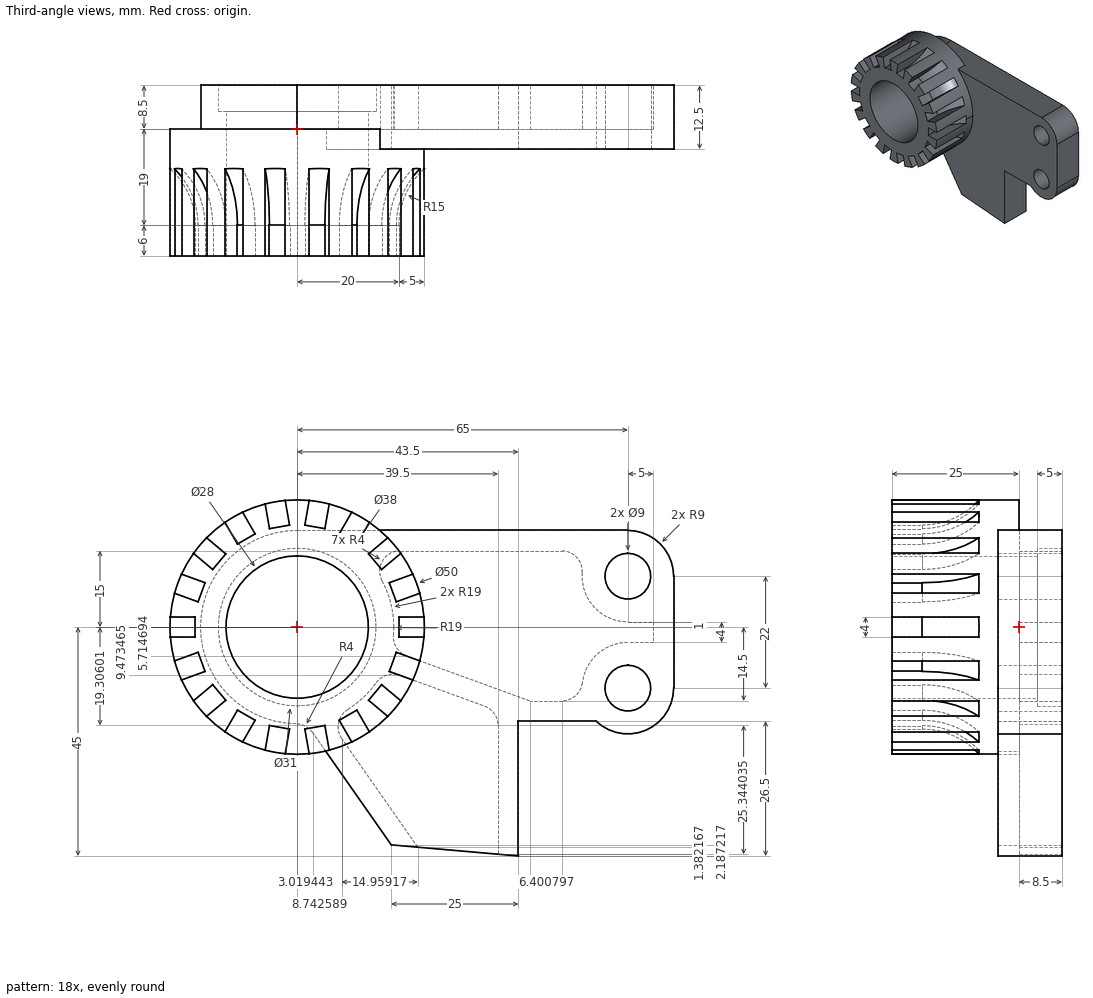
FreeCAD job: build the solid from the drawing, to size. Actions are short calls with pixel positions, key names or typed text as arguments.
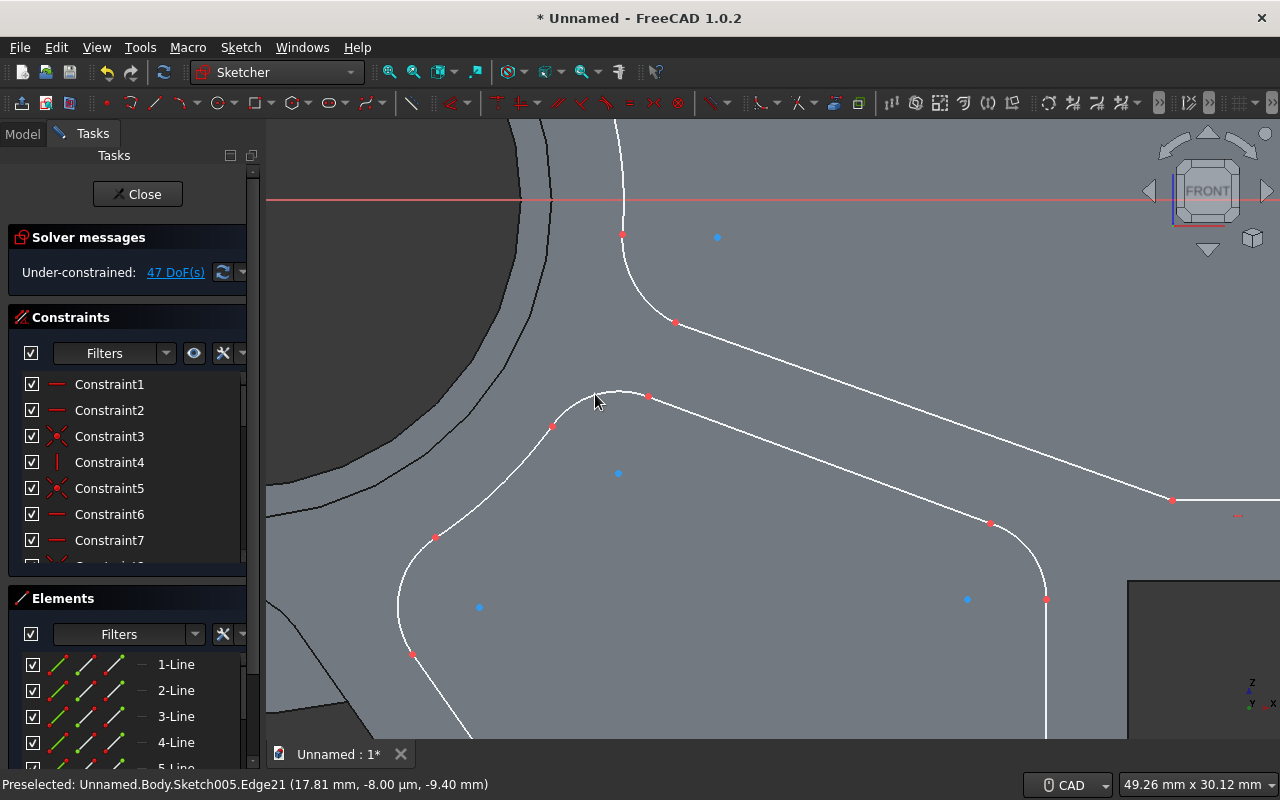
scroll(597, 396, down, 6)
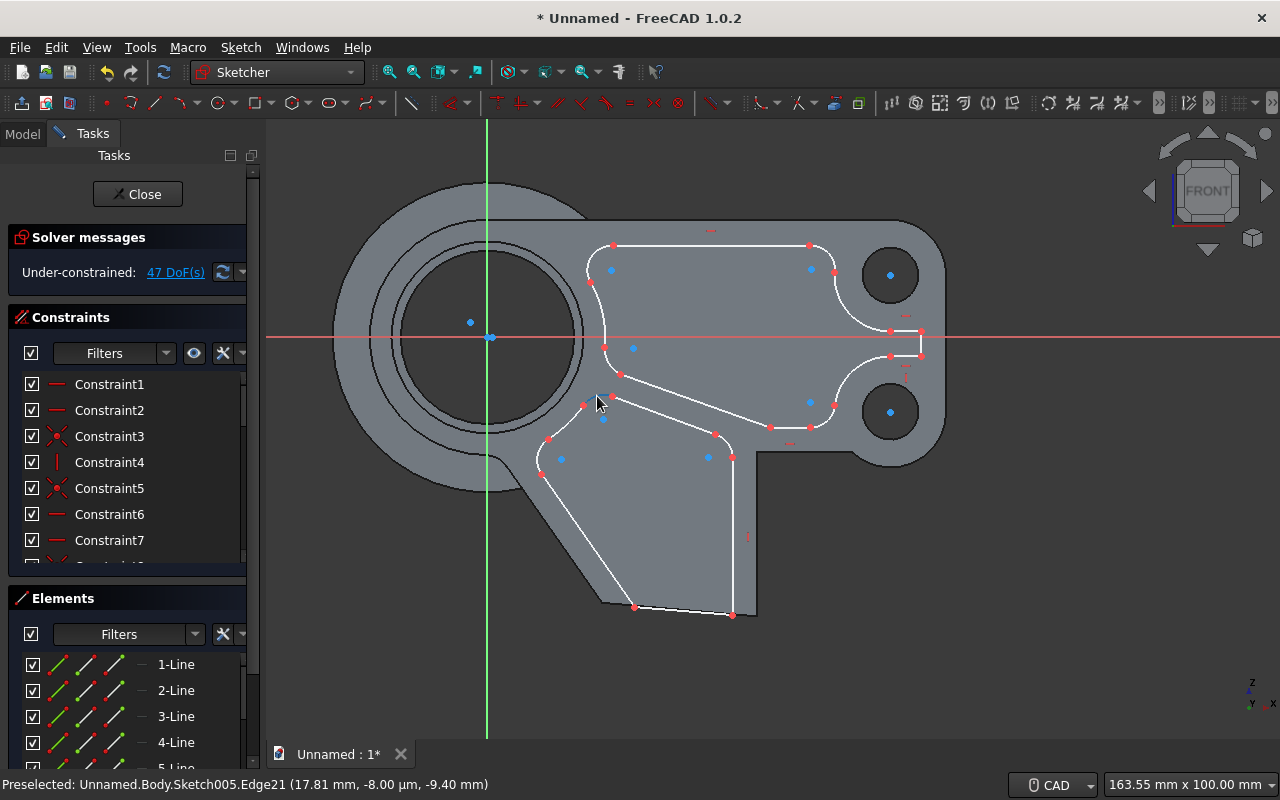
click(672, 246)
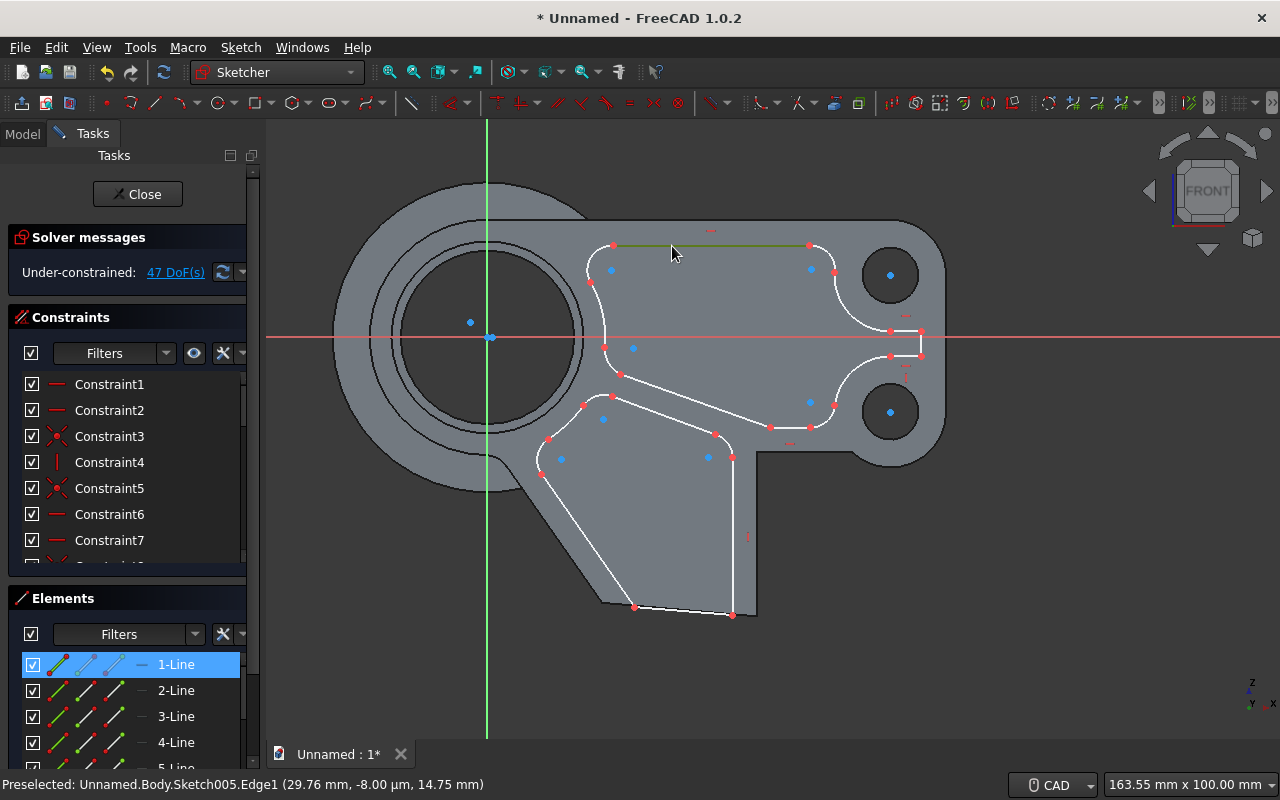
click(833, 260)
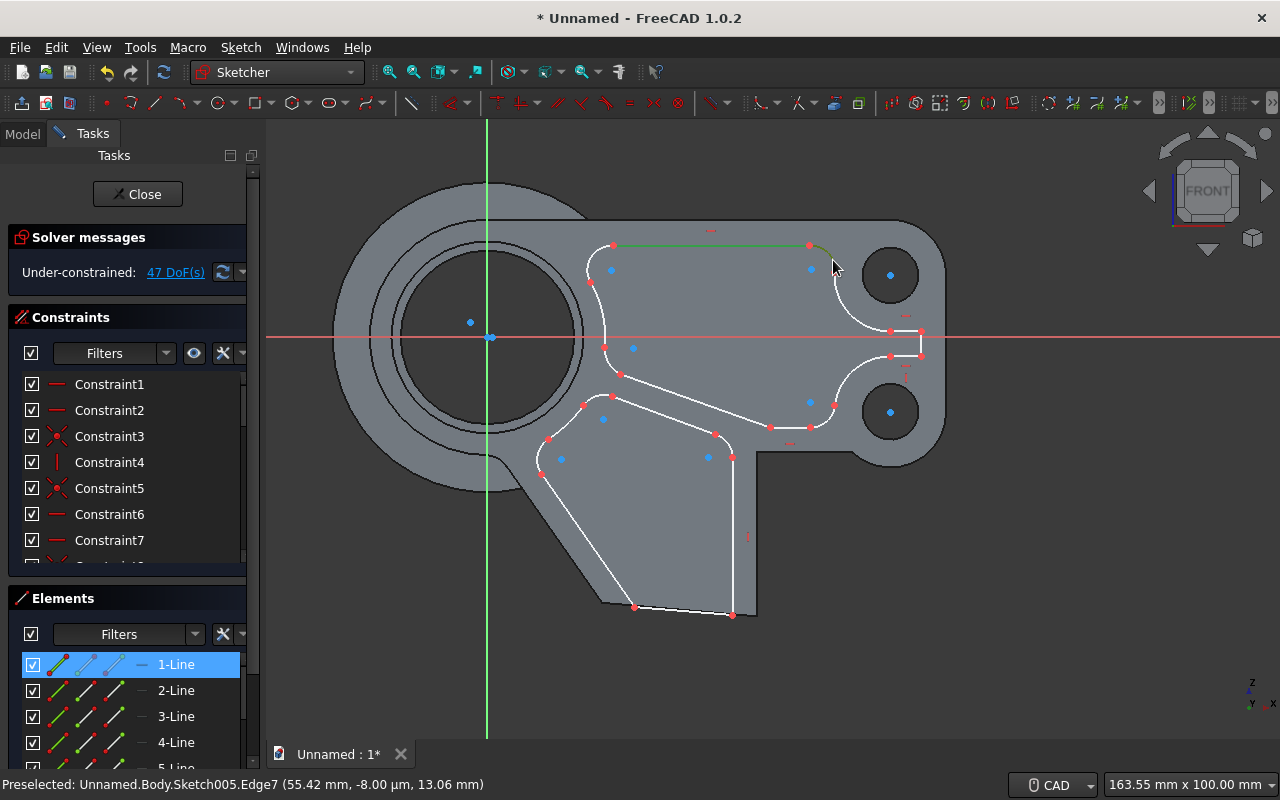
click(606, 104)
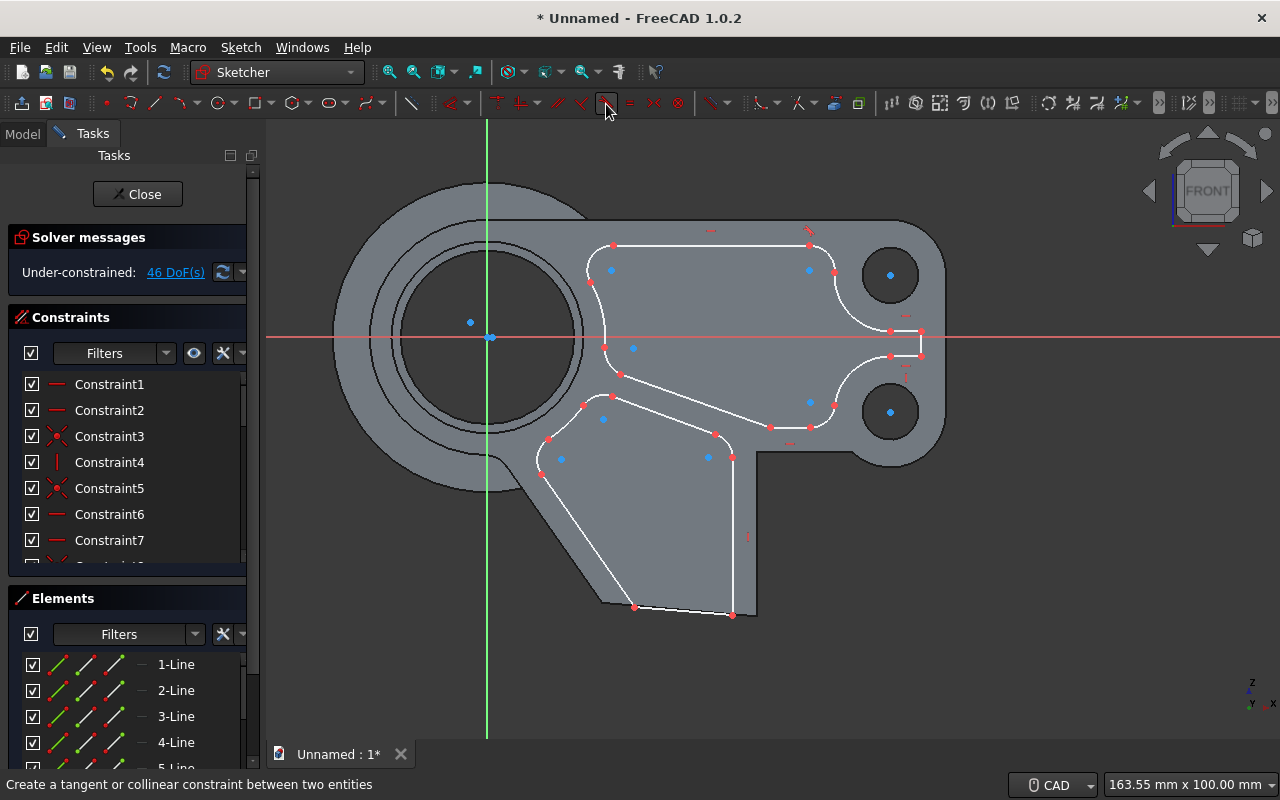
click(672, 246)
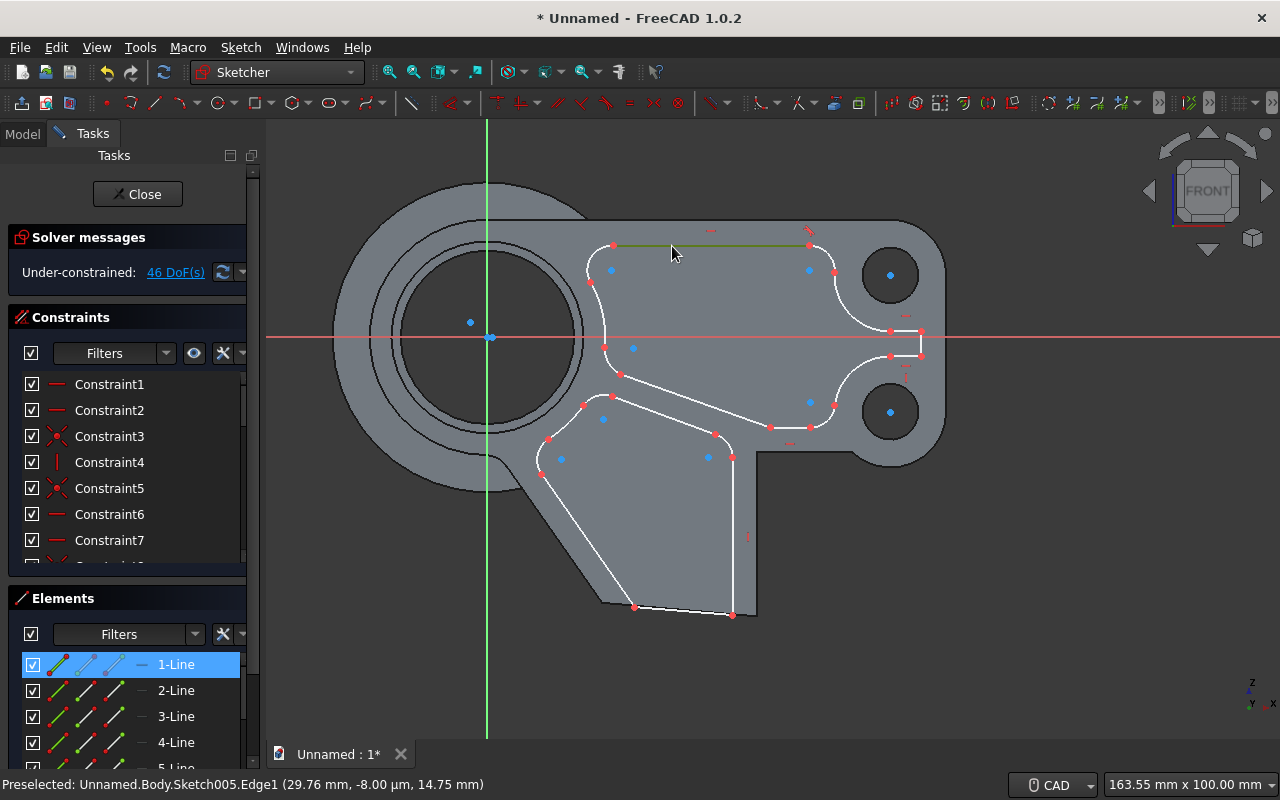
click(598, 250)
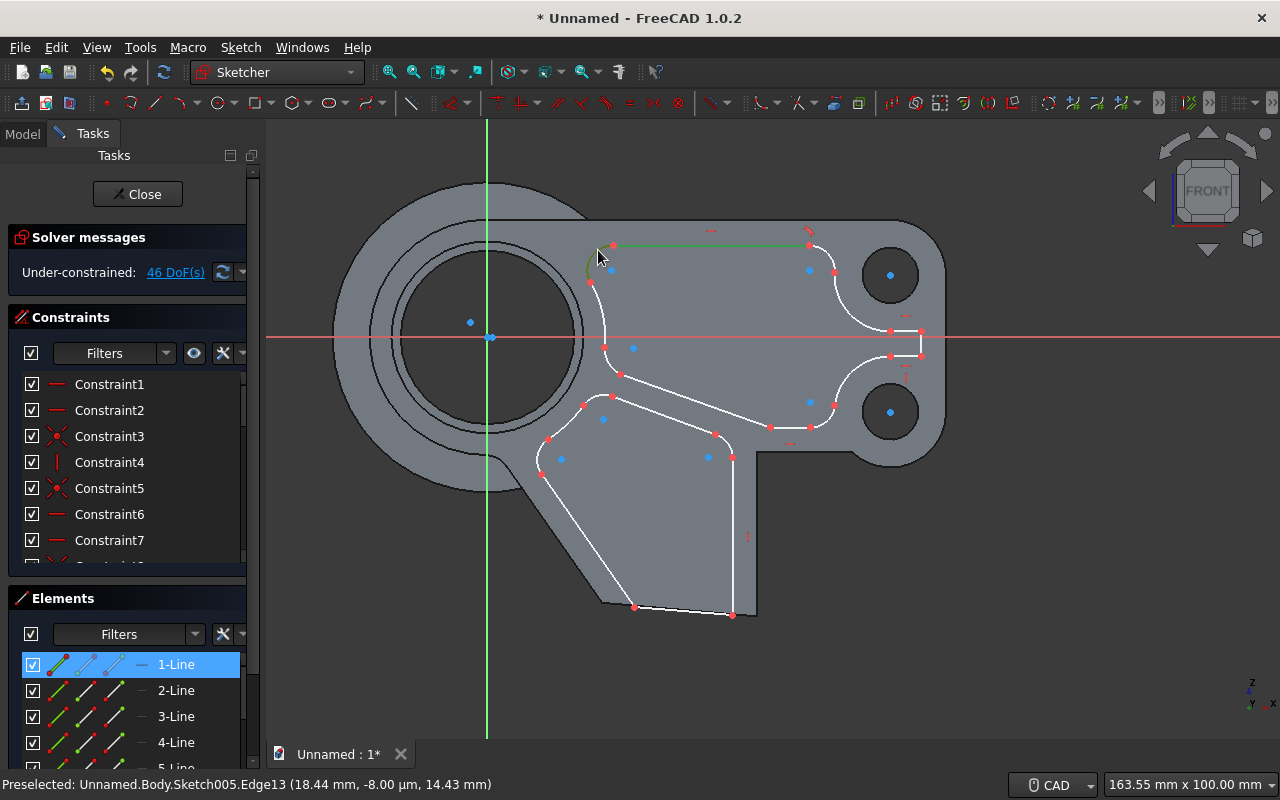
click(606, 104)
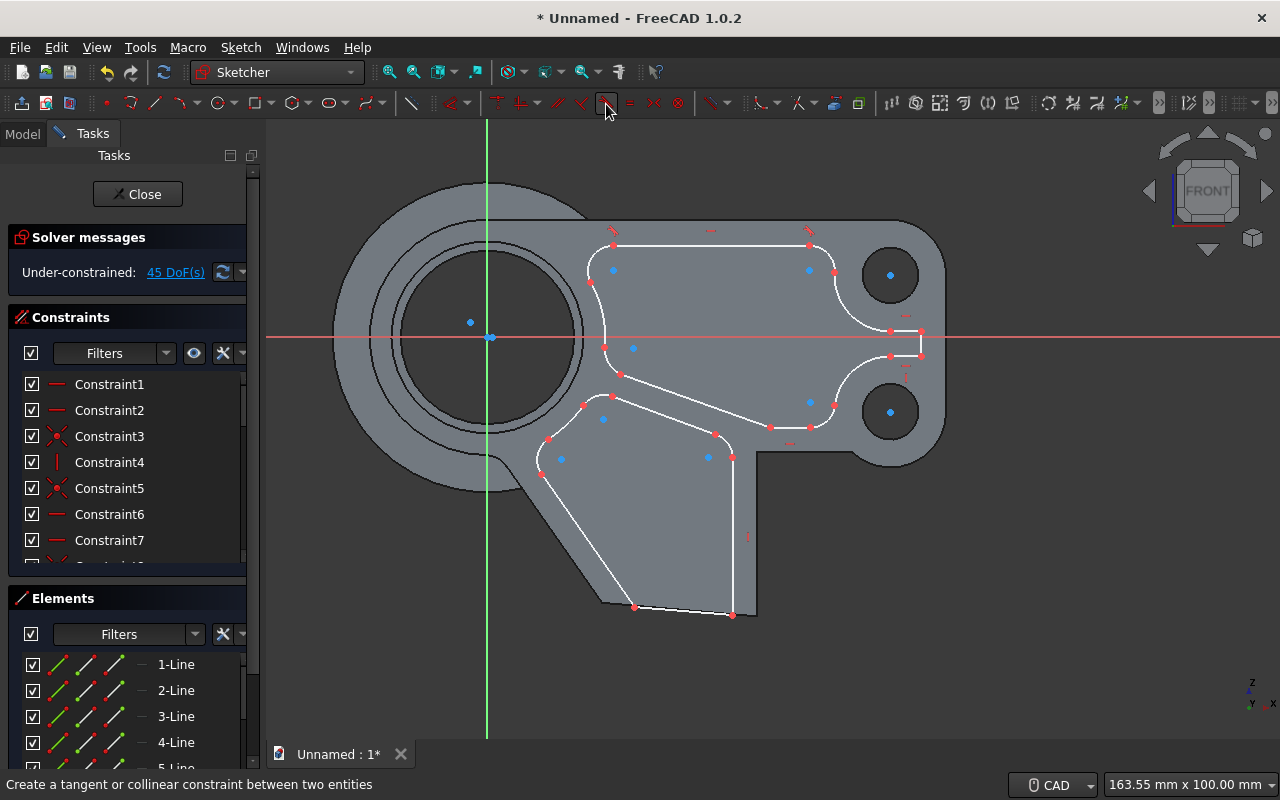
scroll(900, 331, up, 5)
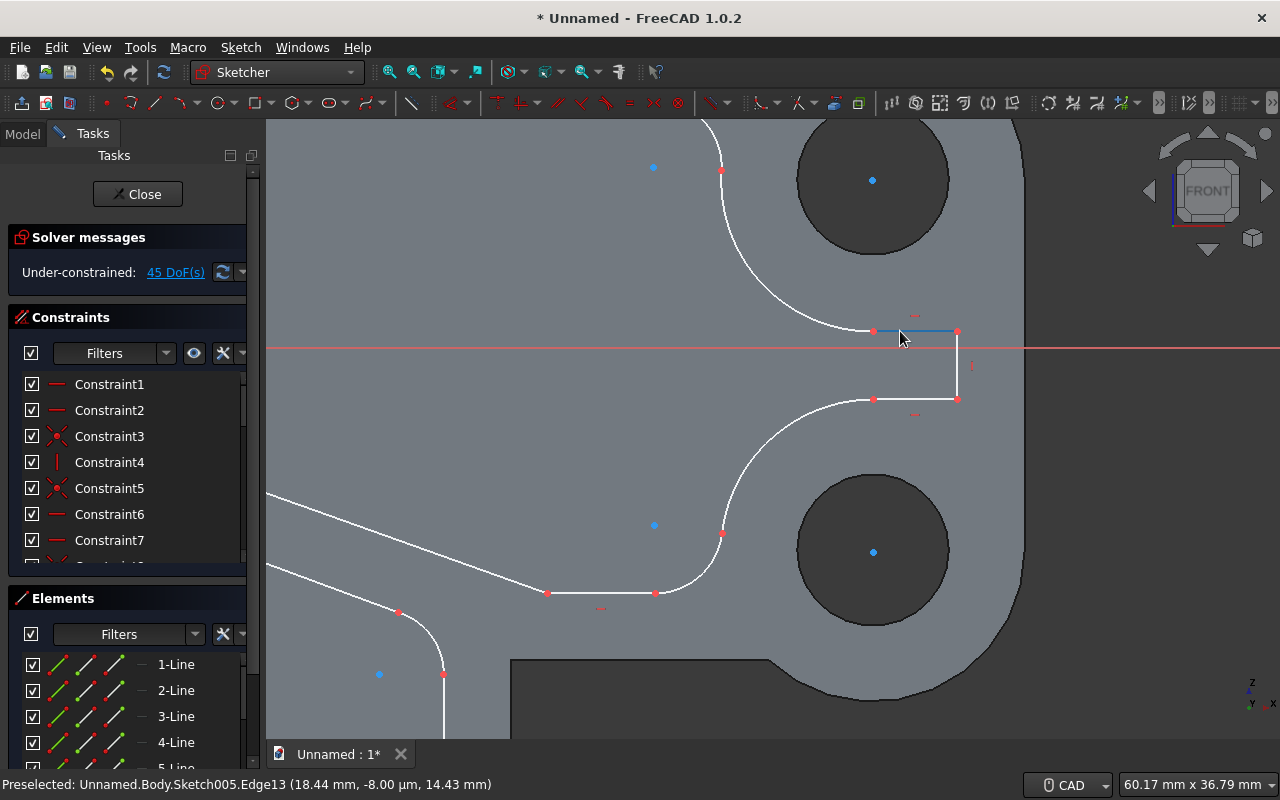
click(899, 331)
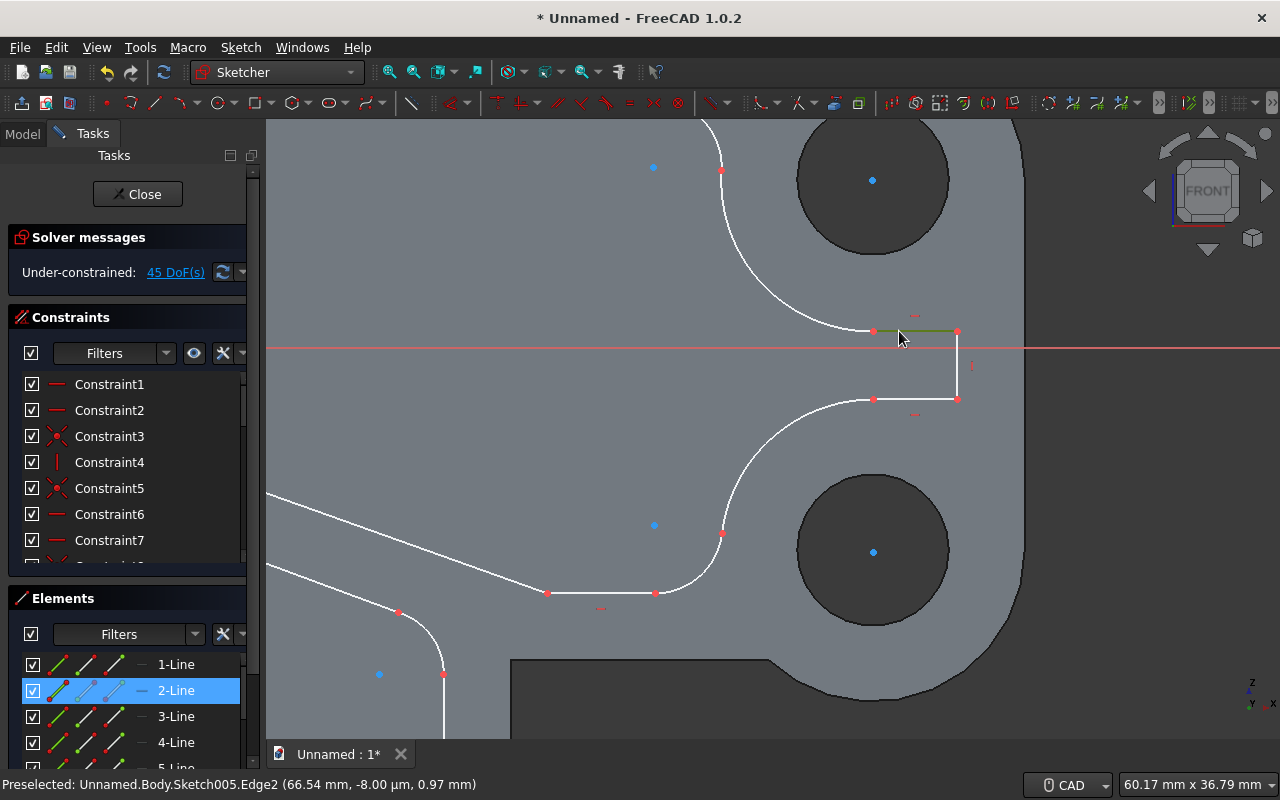
click(735, 243)